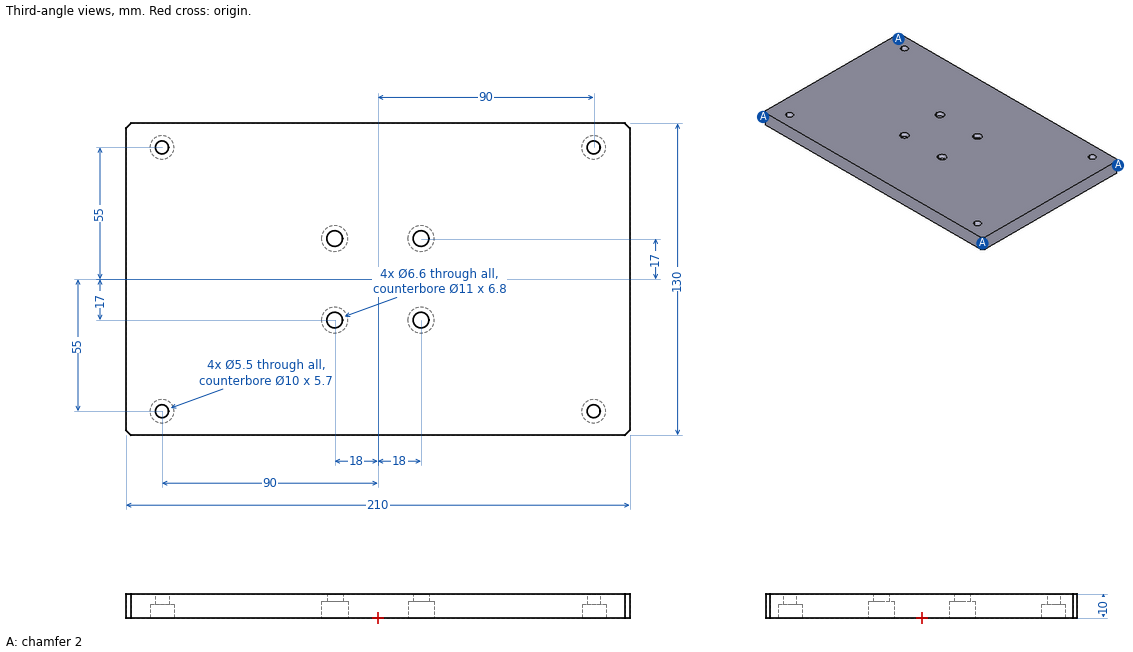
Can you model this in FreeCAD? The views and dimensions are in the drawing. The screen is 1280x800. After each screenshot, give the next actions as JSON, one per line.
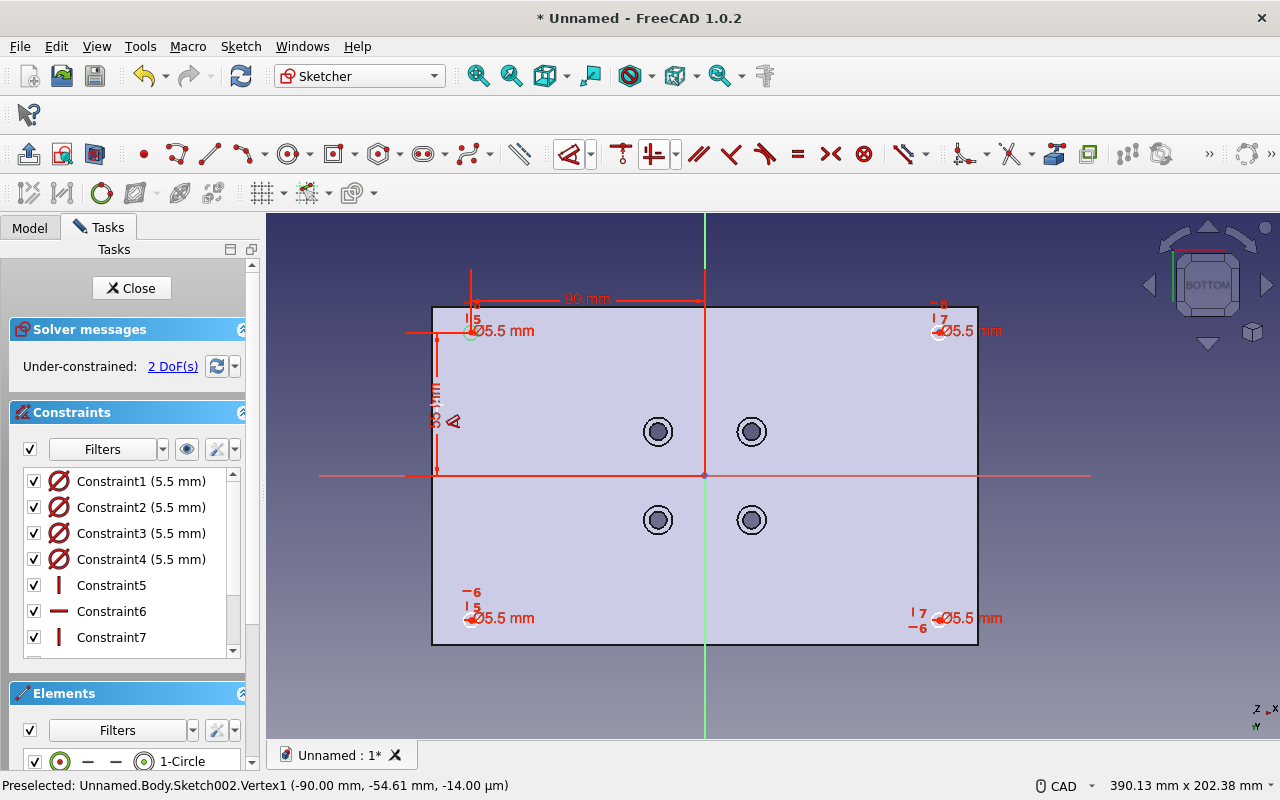
{"action": "left_click", "coordinate": [471, 620]}
{"action": "left_click", "coordinate": [437, 548]}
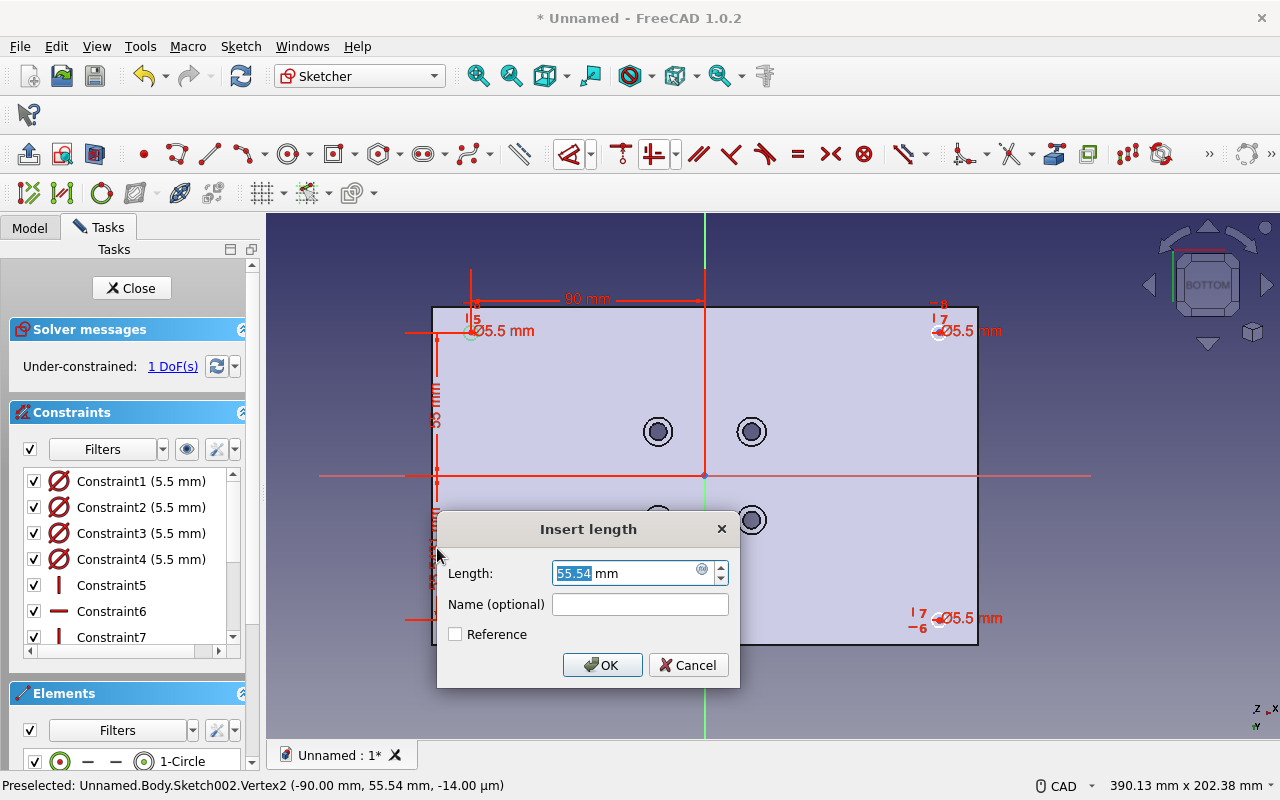
{"action": "type", "text": "55"}
{"action": "key", "text": "Return"}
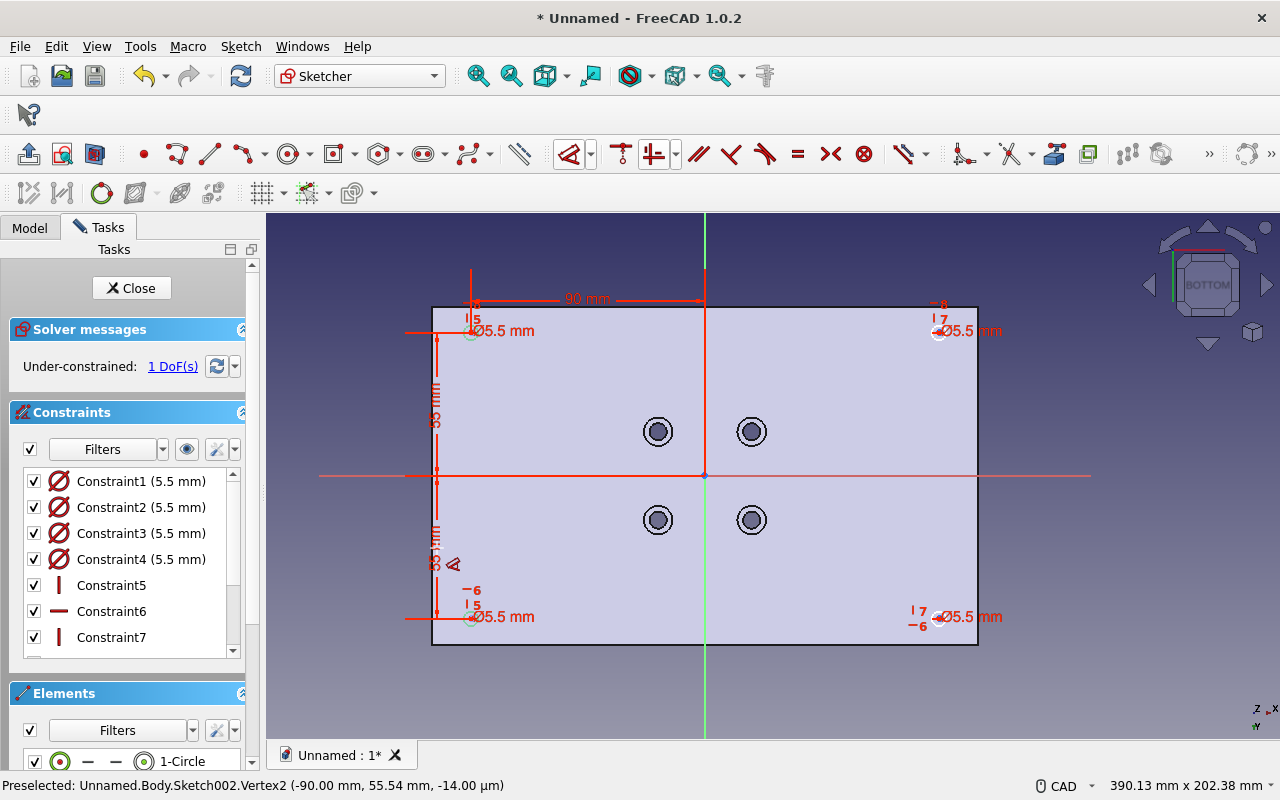
{"action": "left_click", "coordinate": [939, 619]}
{"action": "left_click", "coordinate": [822, 653]}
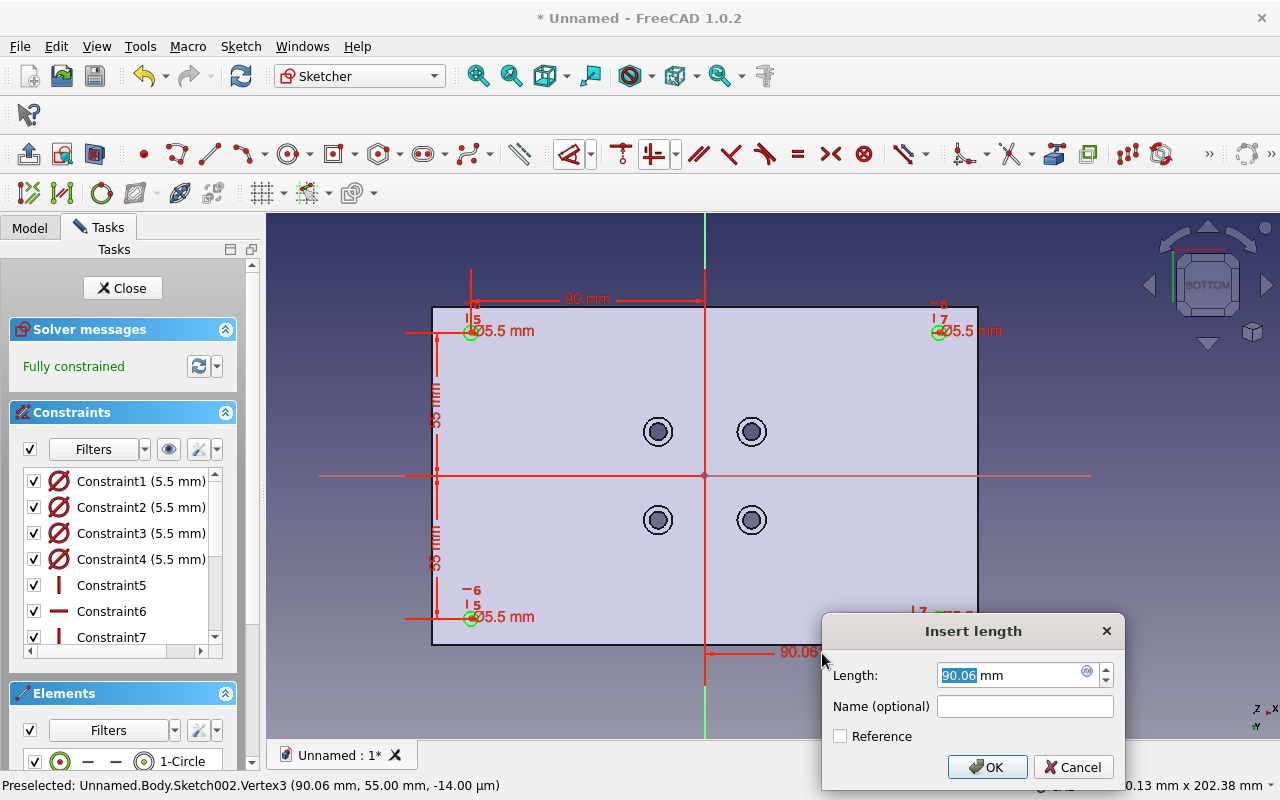
{"action": "type", "text": "90"}
{"action": "key", "text": "Return"}
{"action": "key", "text": "Escape"}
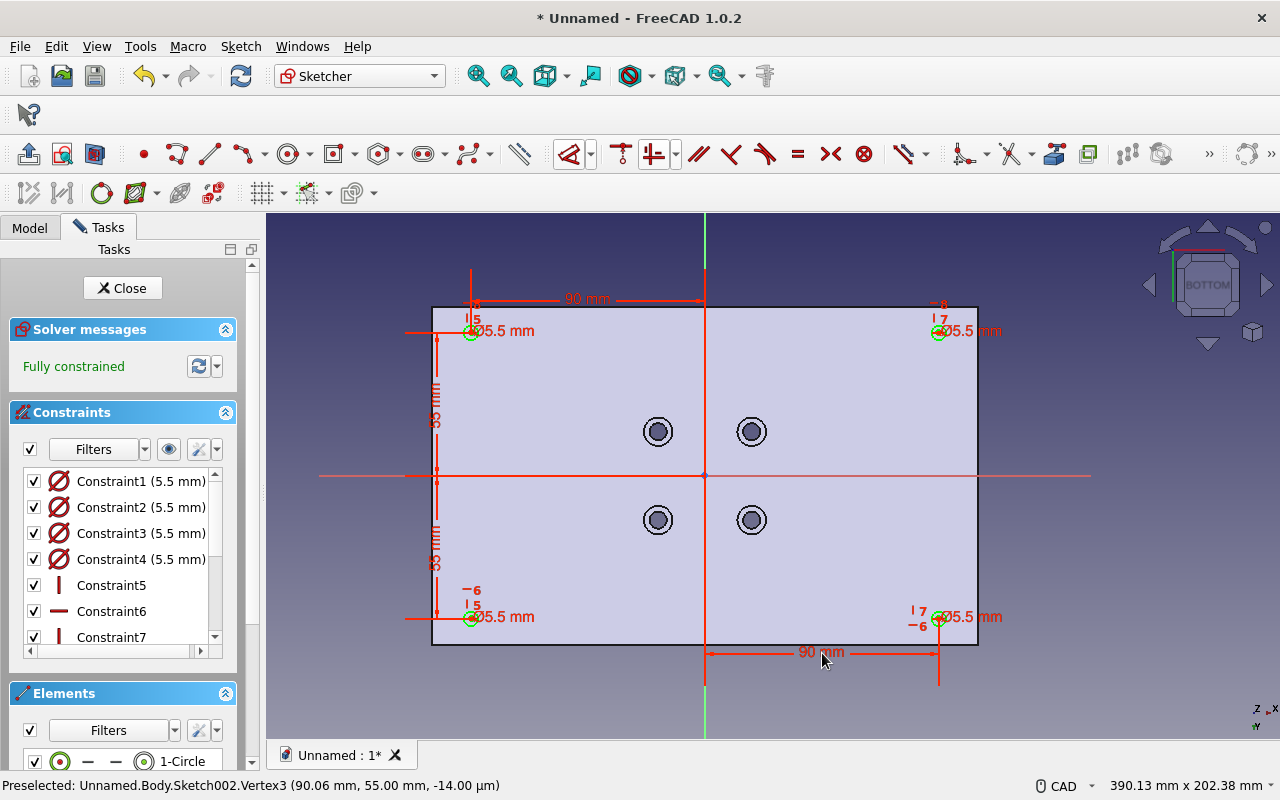
{"action": "left_click", "coordinate": [123, 288]}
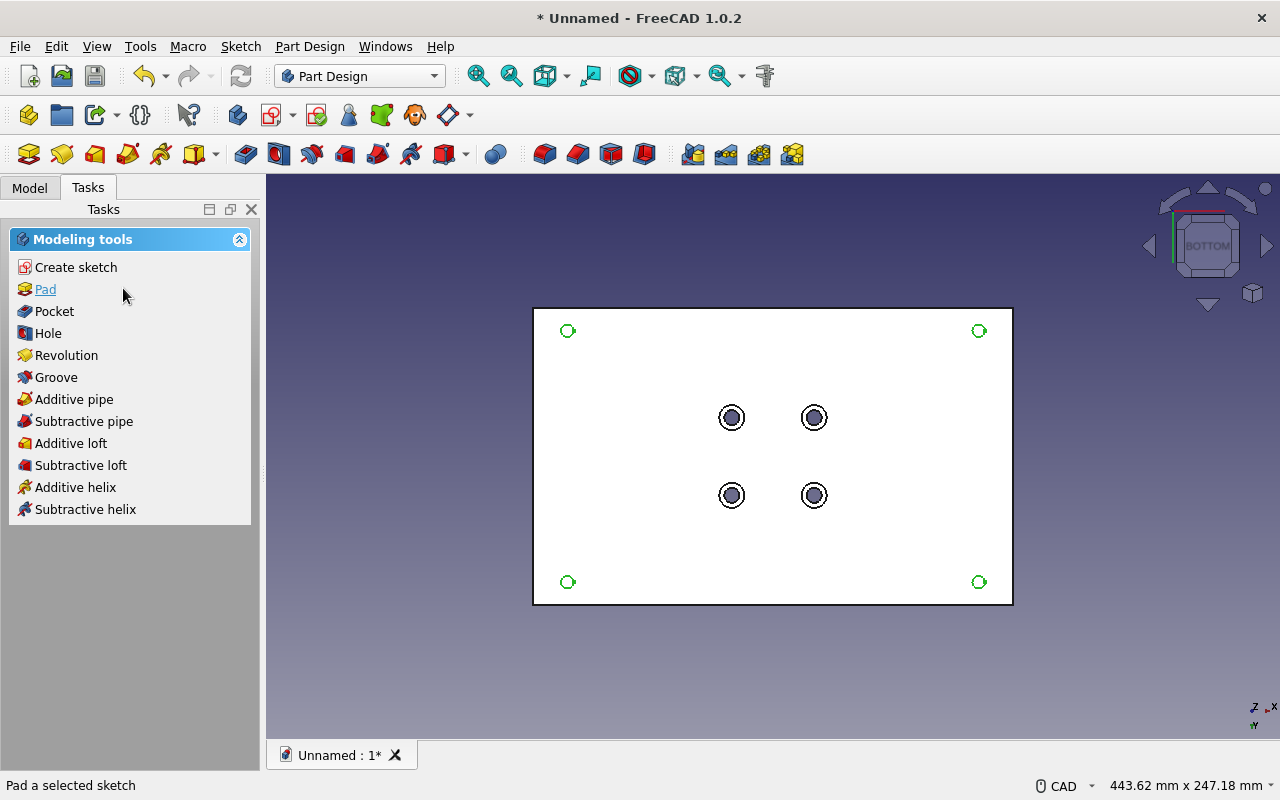
{"action": "left_click", "coordinate": [279, 154]}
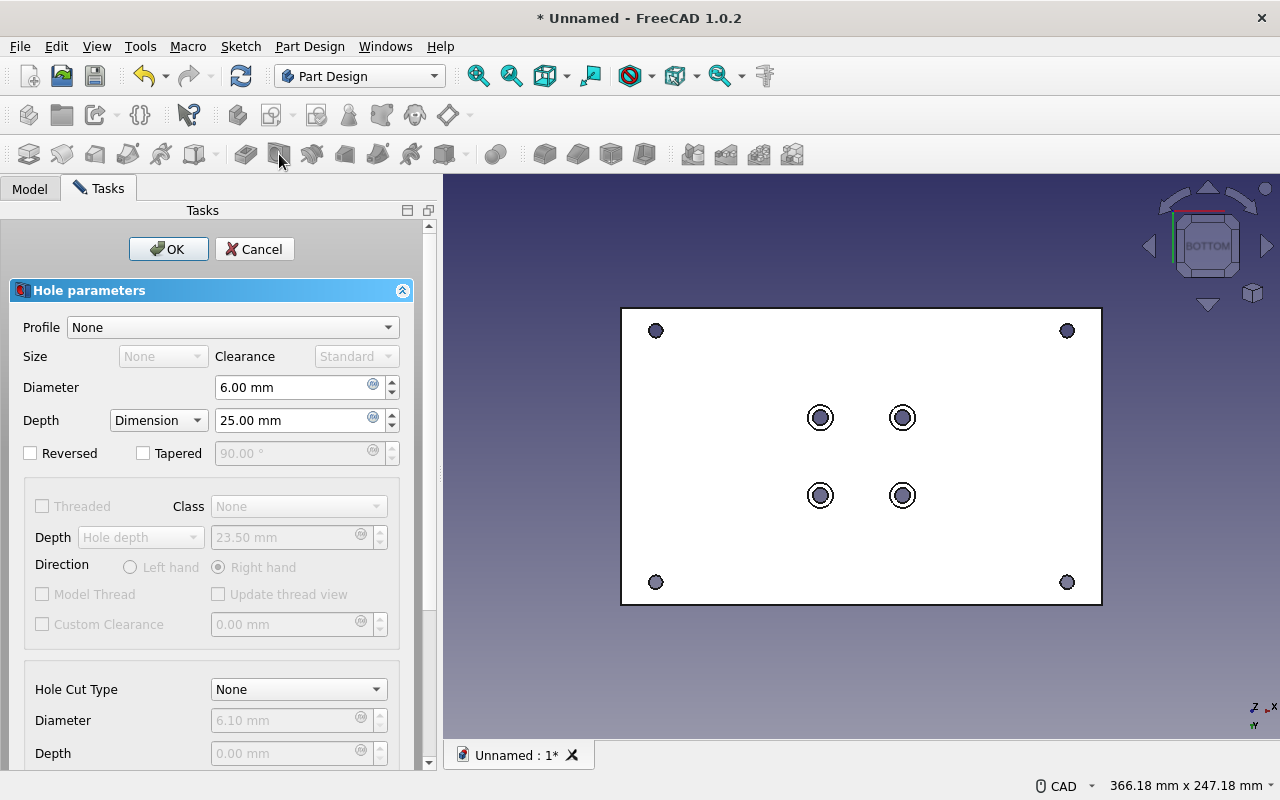
{"action": "triple_click", "coordinate": [300, 388]}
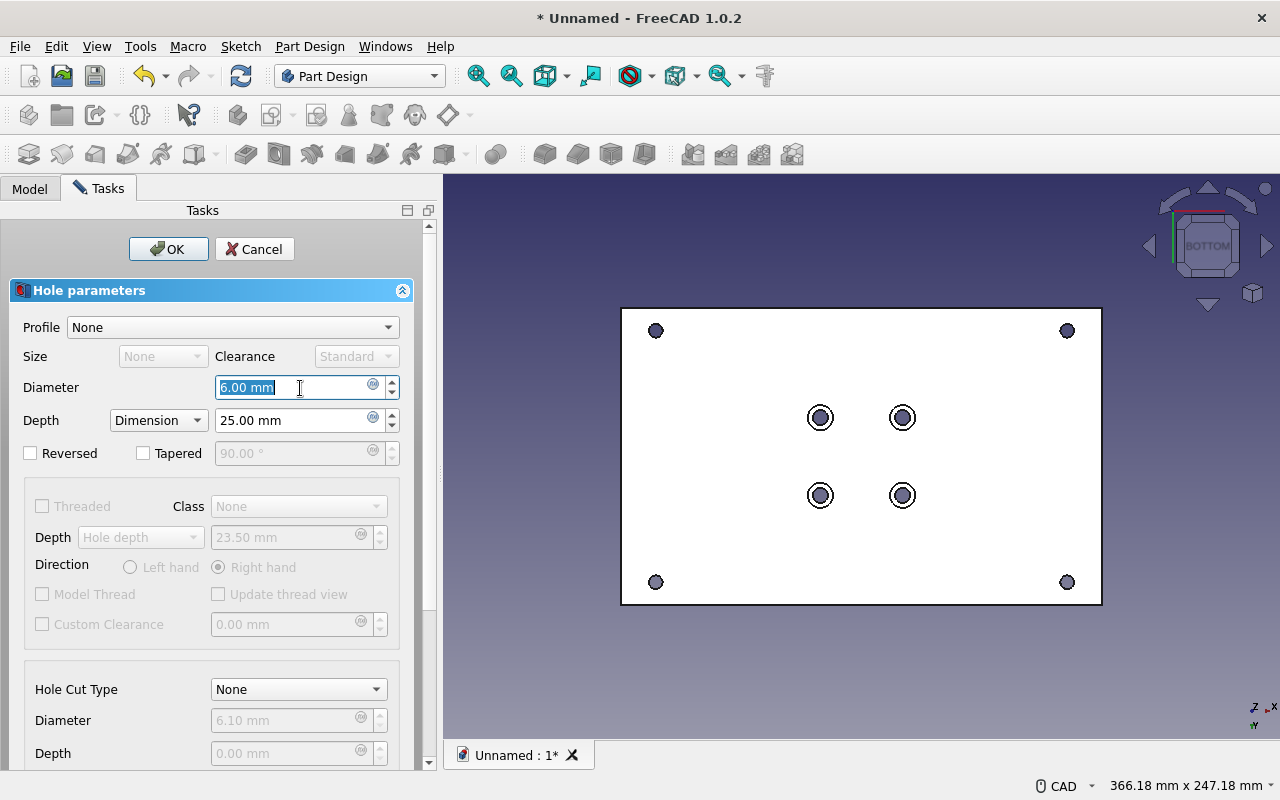
{"action": "type", "text": "5.5"}
{"action": "key", "text": "Tab"}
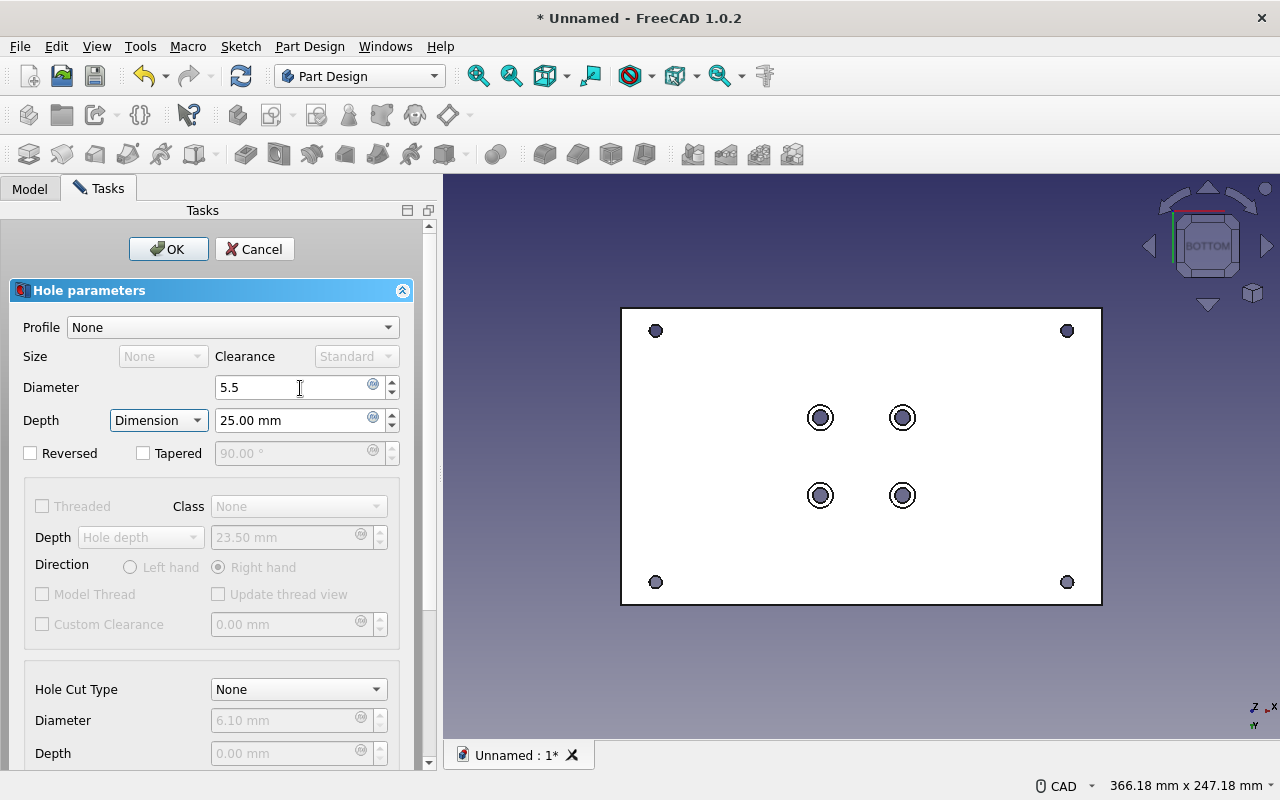
{"action": "left_click", "coordinate": [160, 420]}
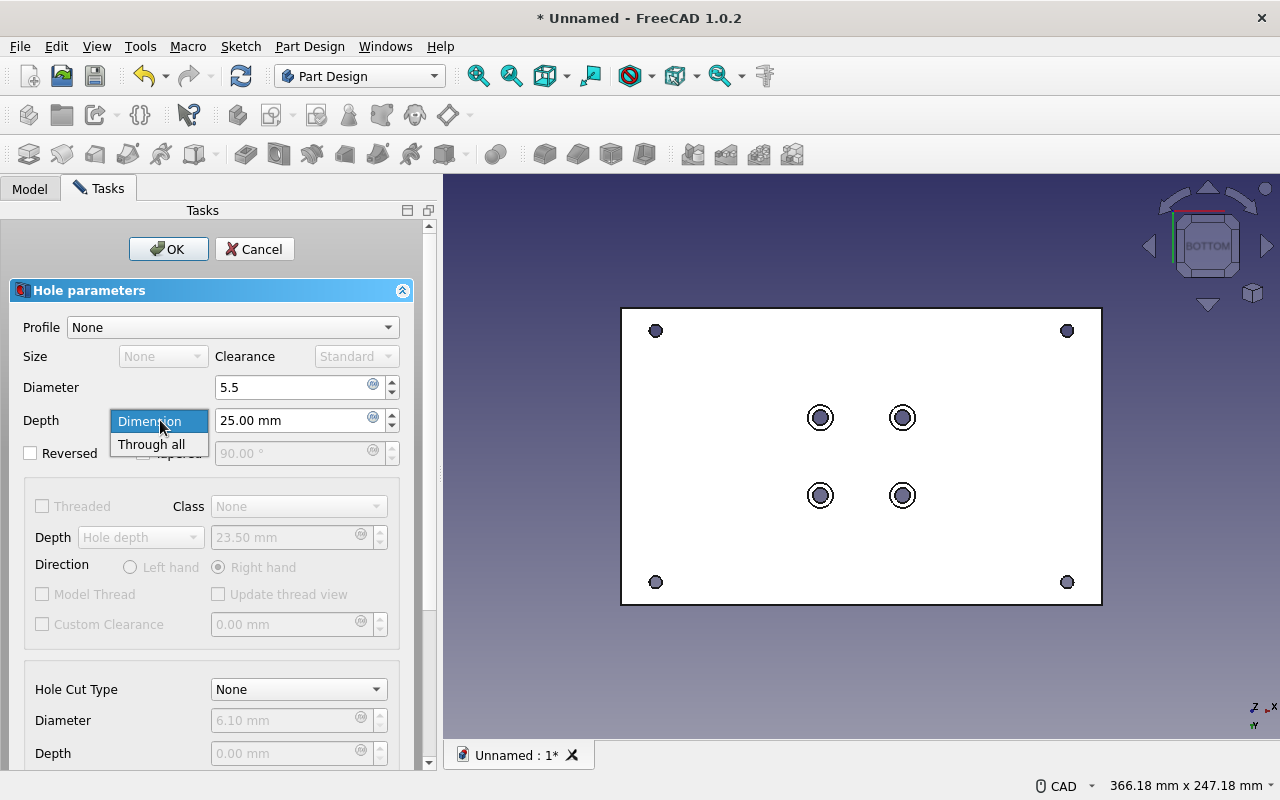
{"action": "left_click", "coordinate": [158, 444]}